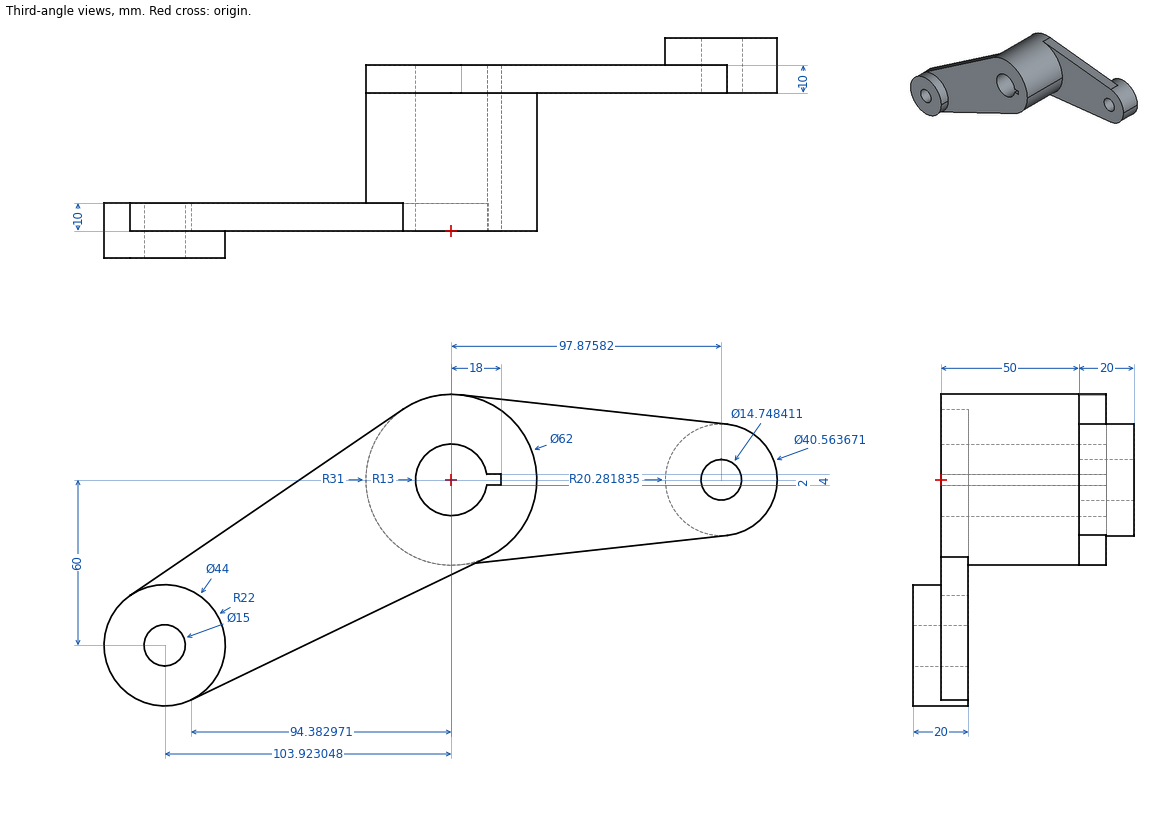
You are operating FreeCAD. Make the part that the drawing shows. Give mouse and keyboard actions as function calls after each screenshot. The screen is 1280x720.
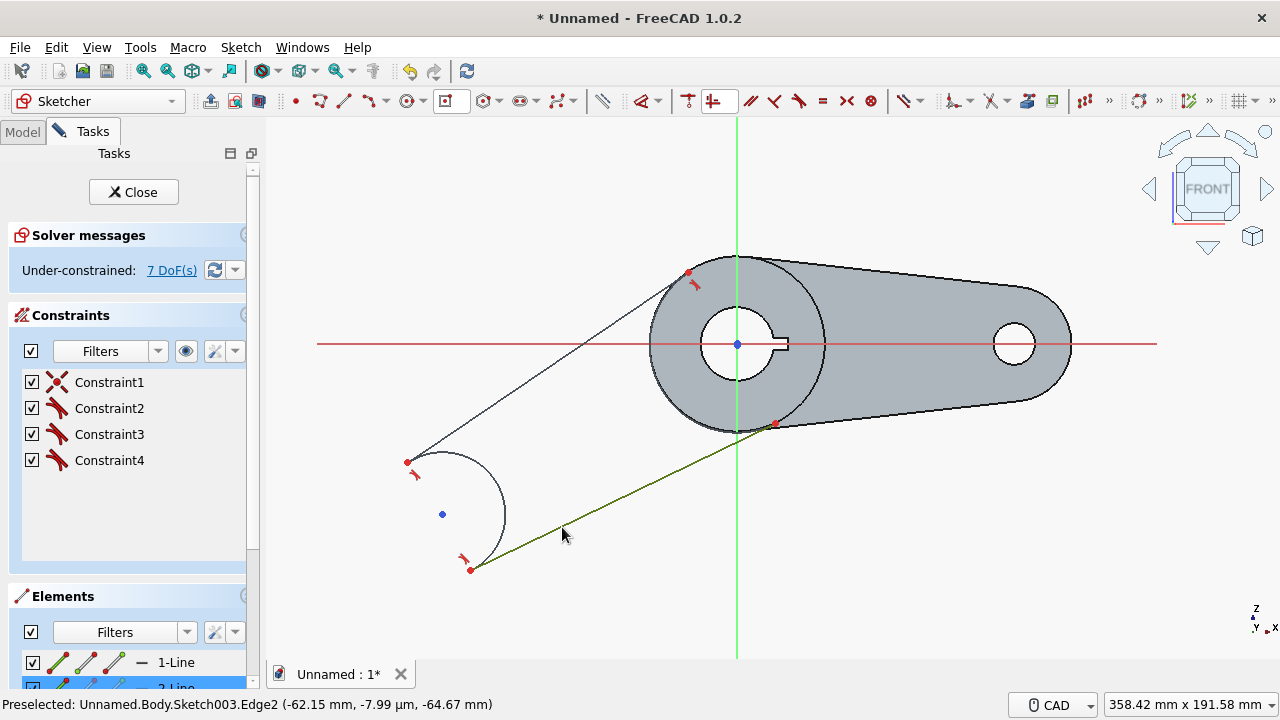
click(699, 424)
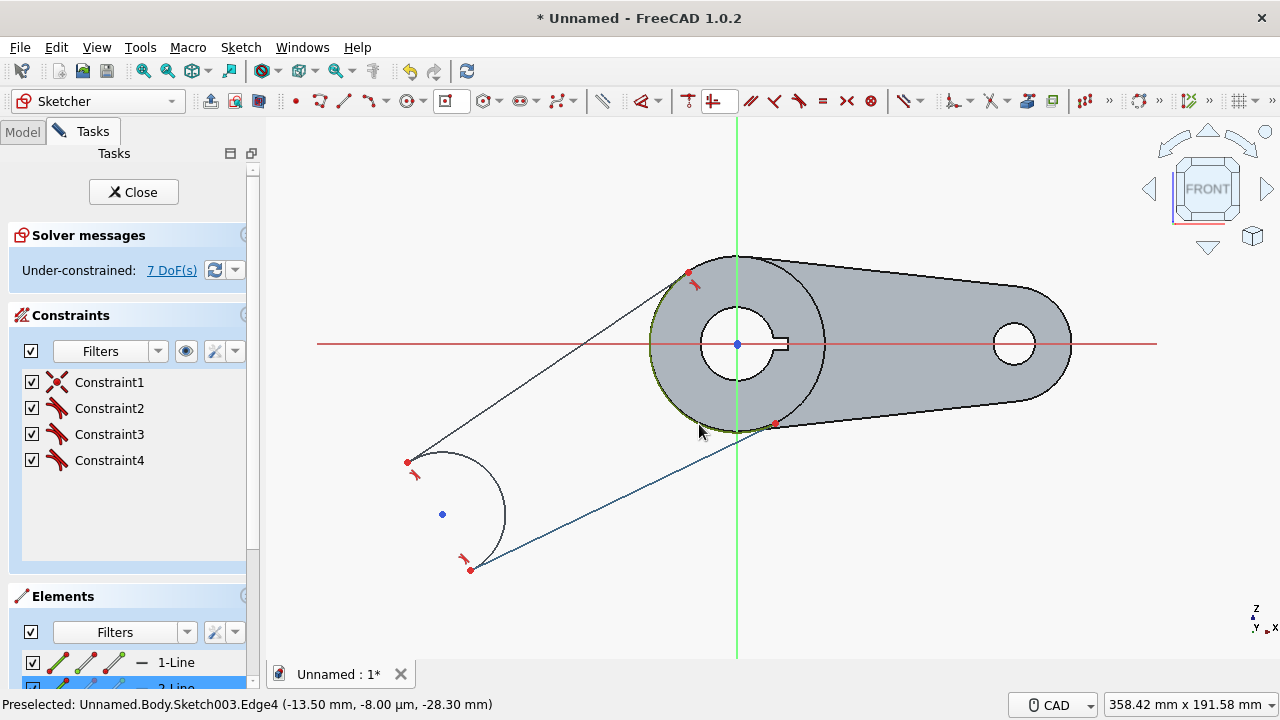
click(800, 102)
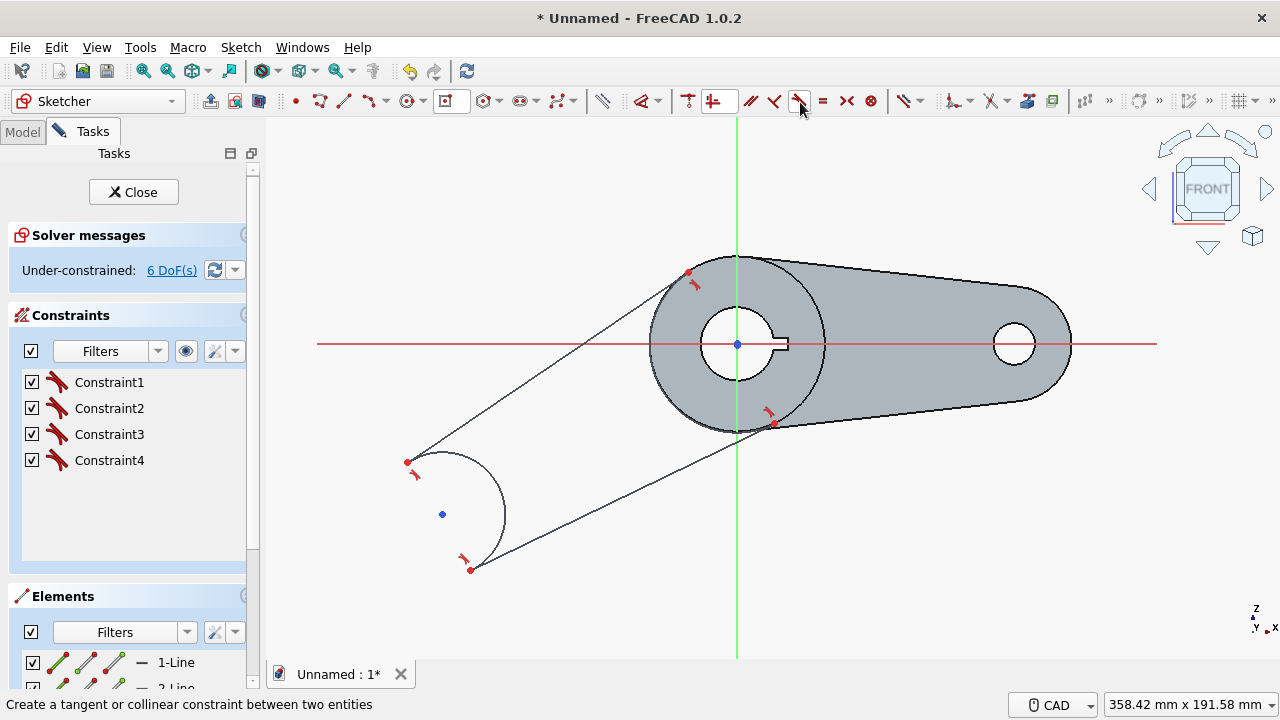
drag(727, 334, 747, 355)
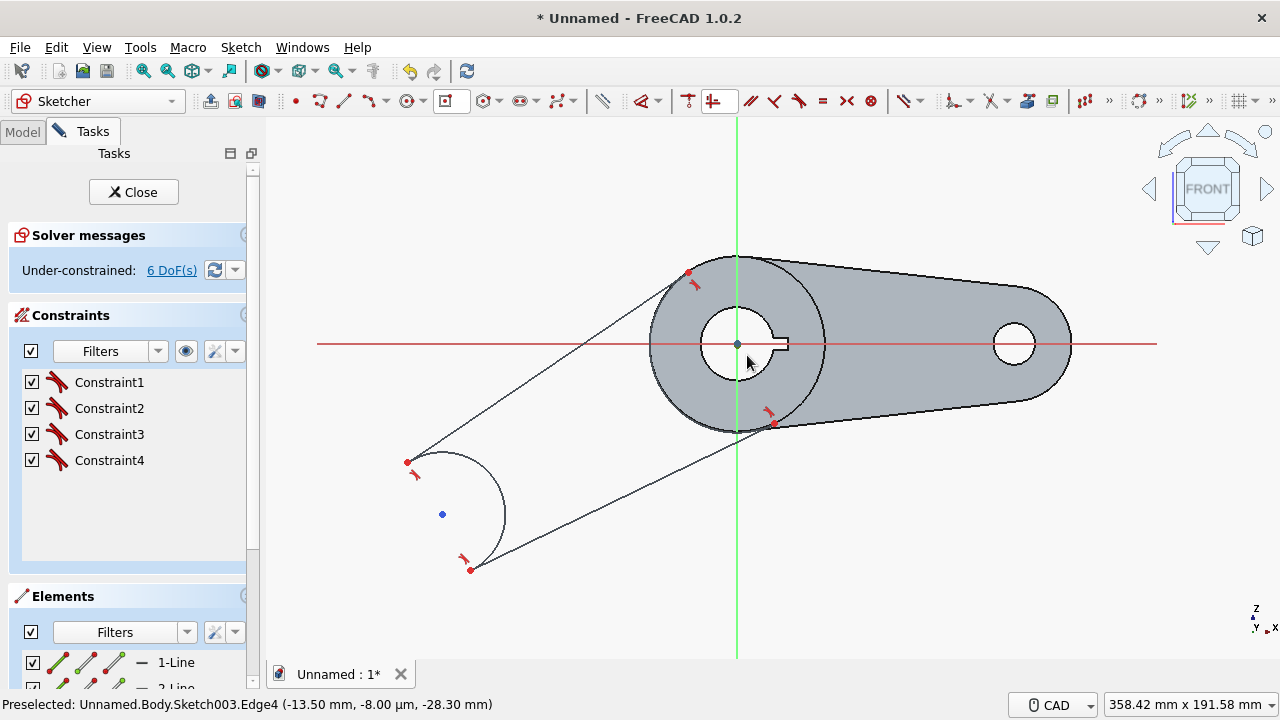
click(688, 102)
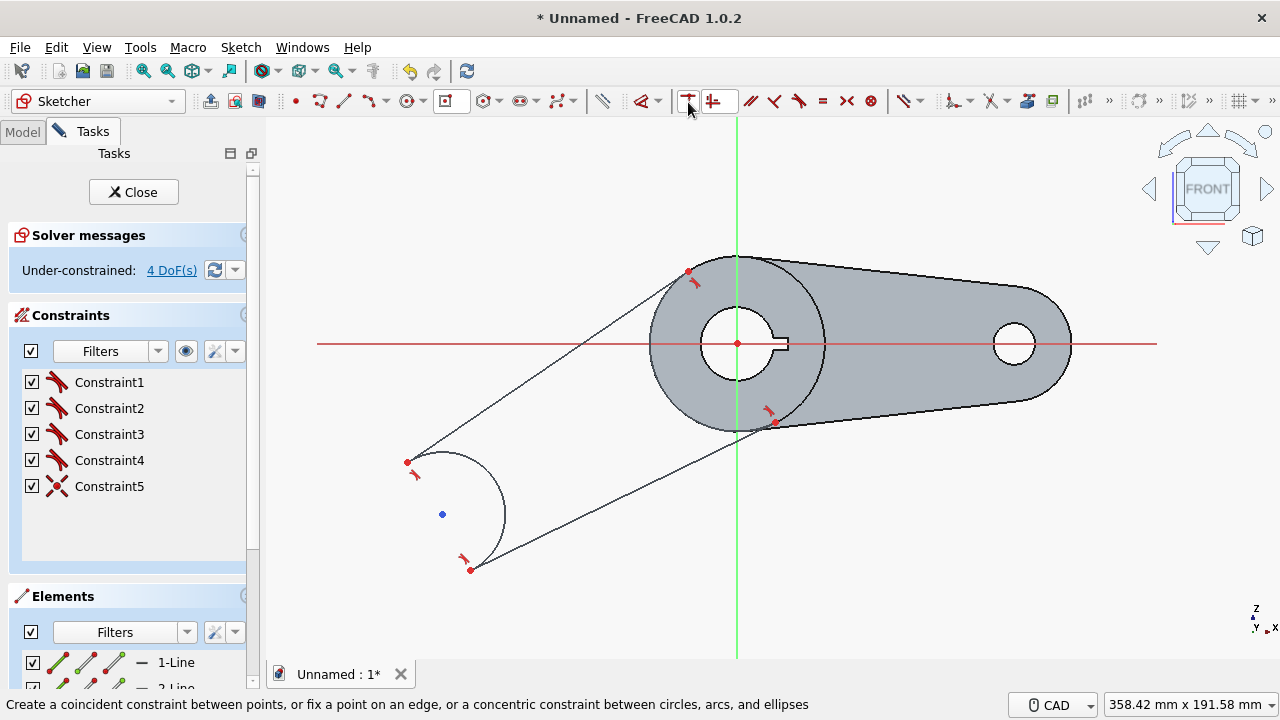
click(642, 102)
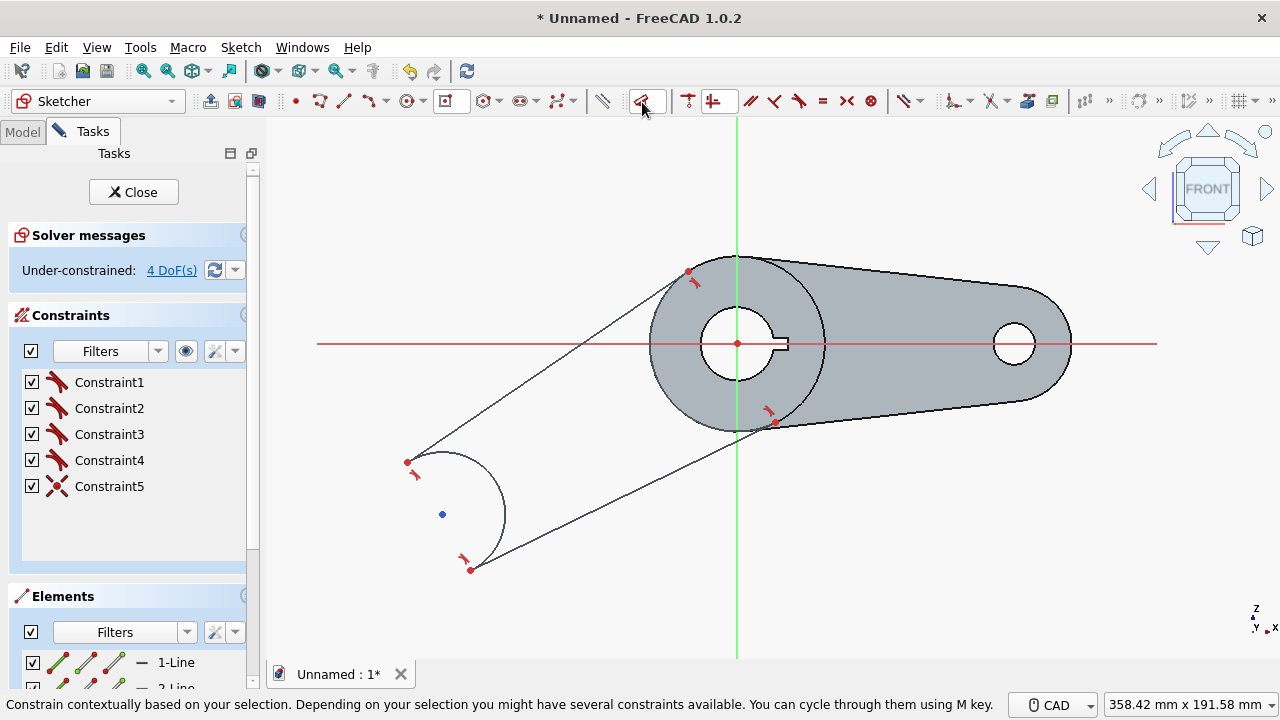
click(505, 523)
click(519, 571)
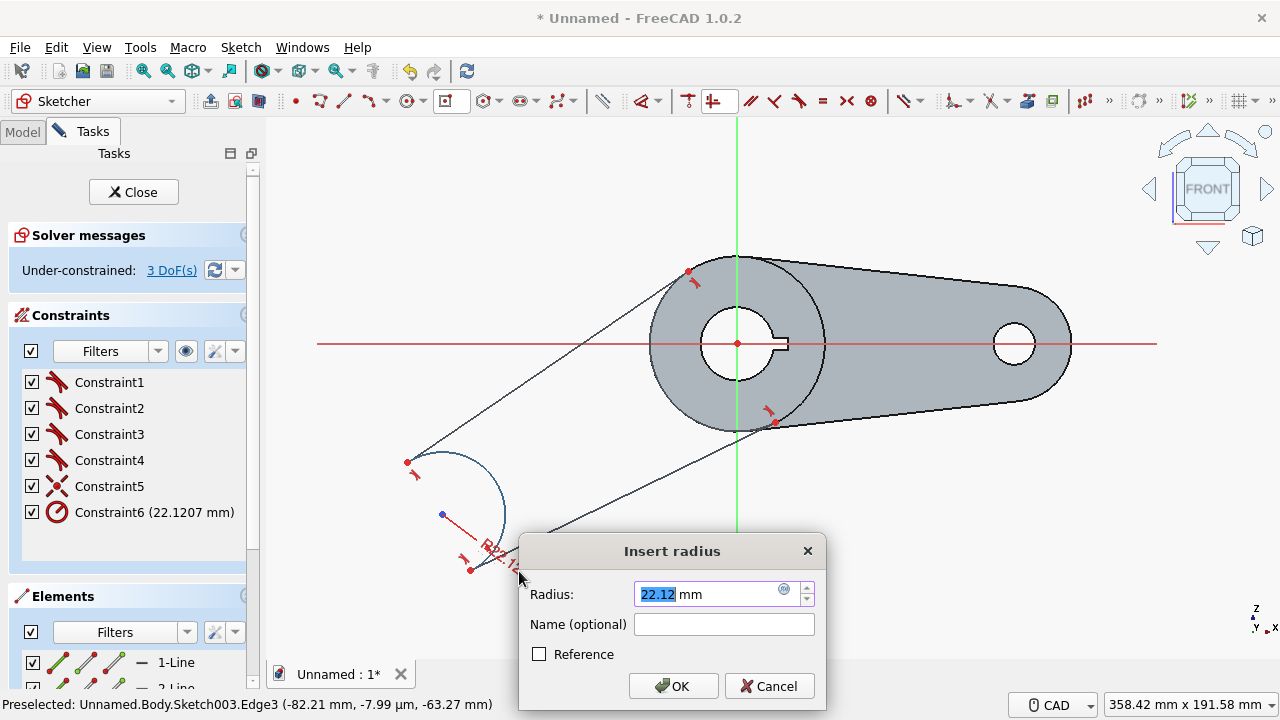
text(22)
key(Return)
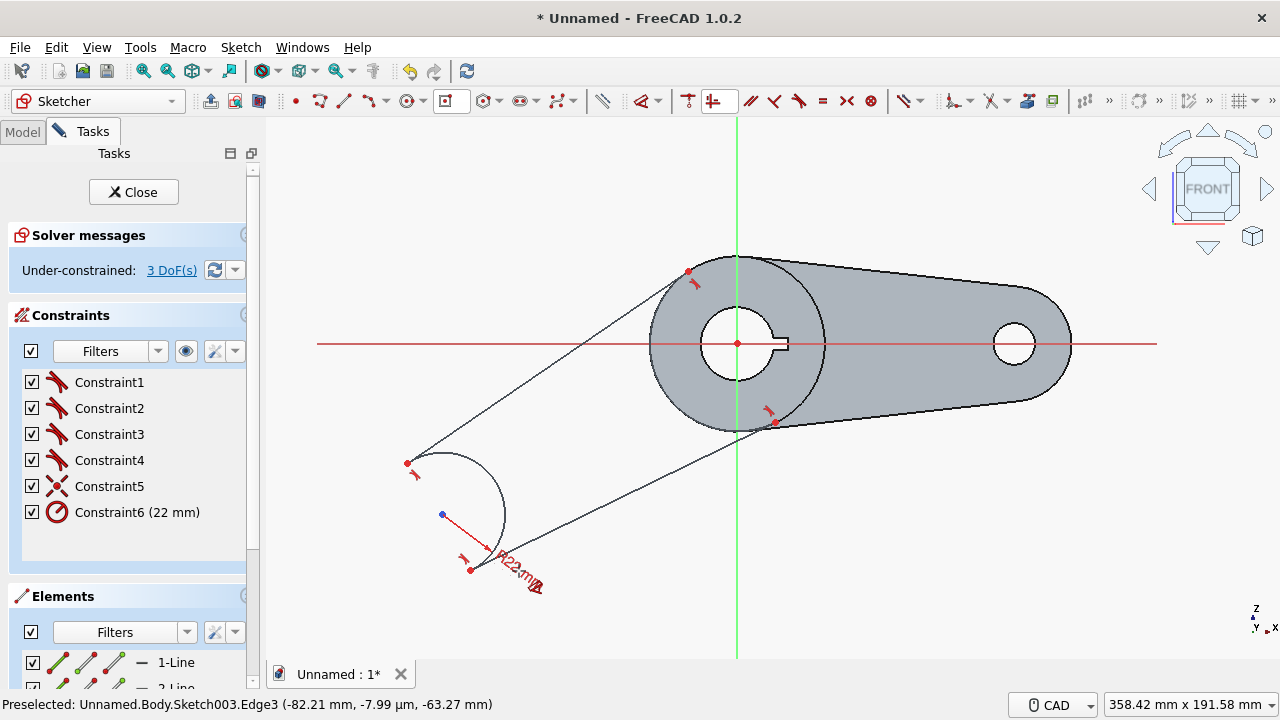
click(700, 423)
click(641, 414)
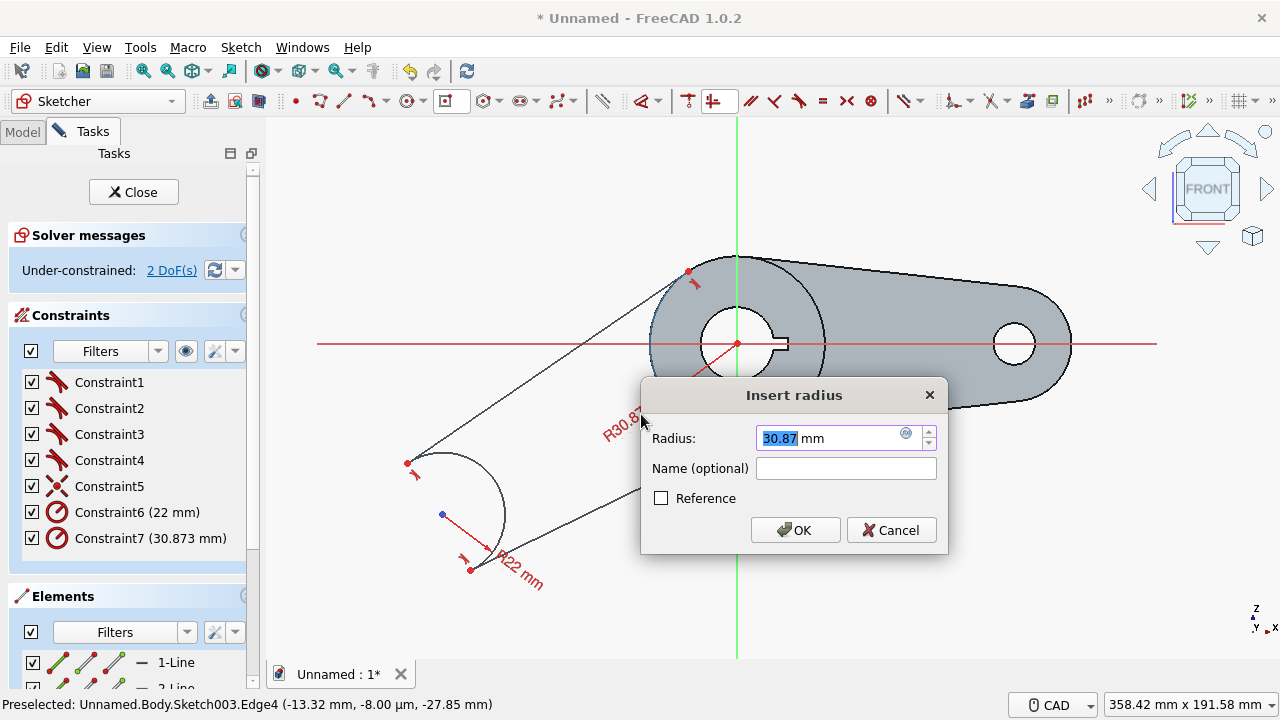
text(31)
key(Return)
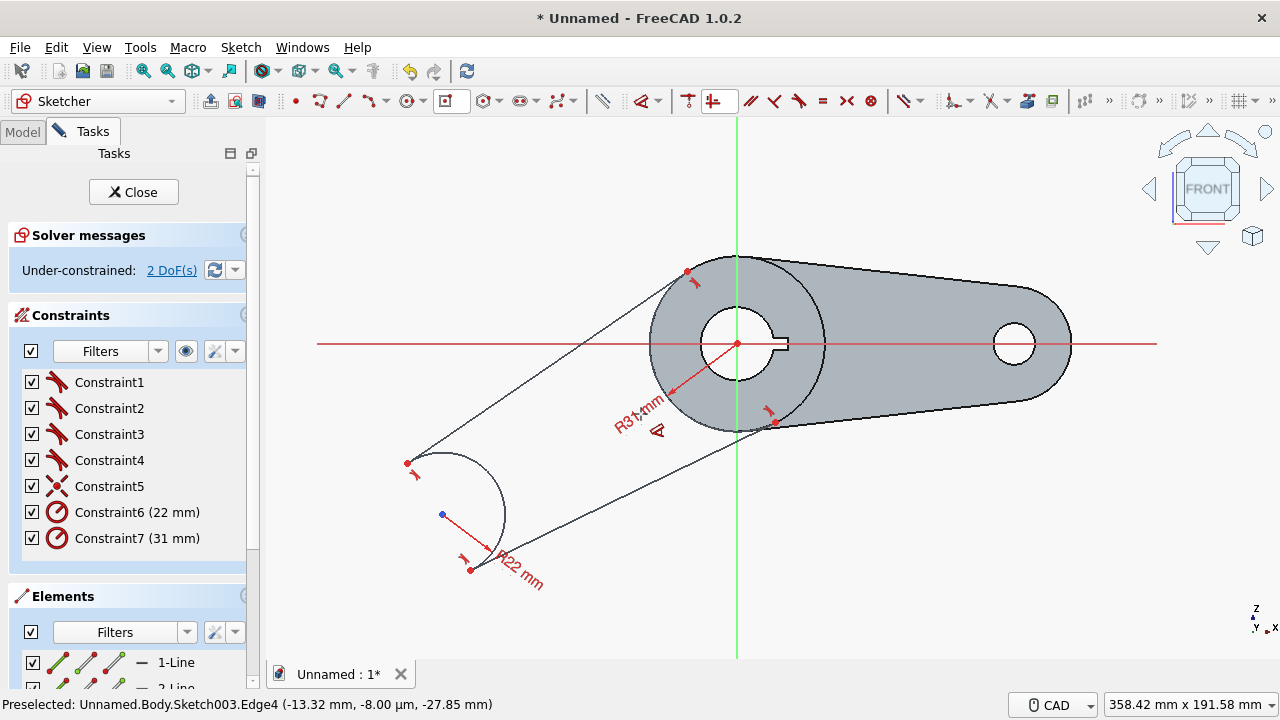
click(443, 515)
click(409, 429)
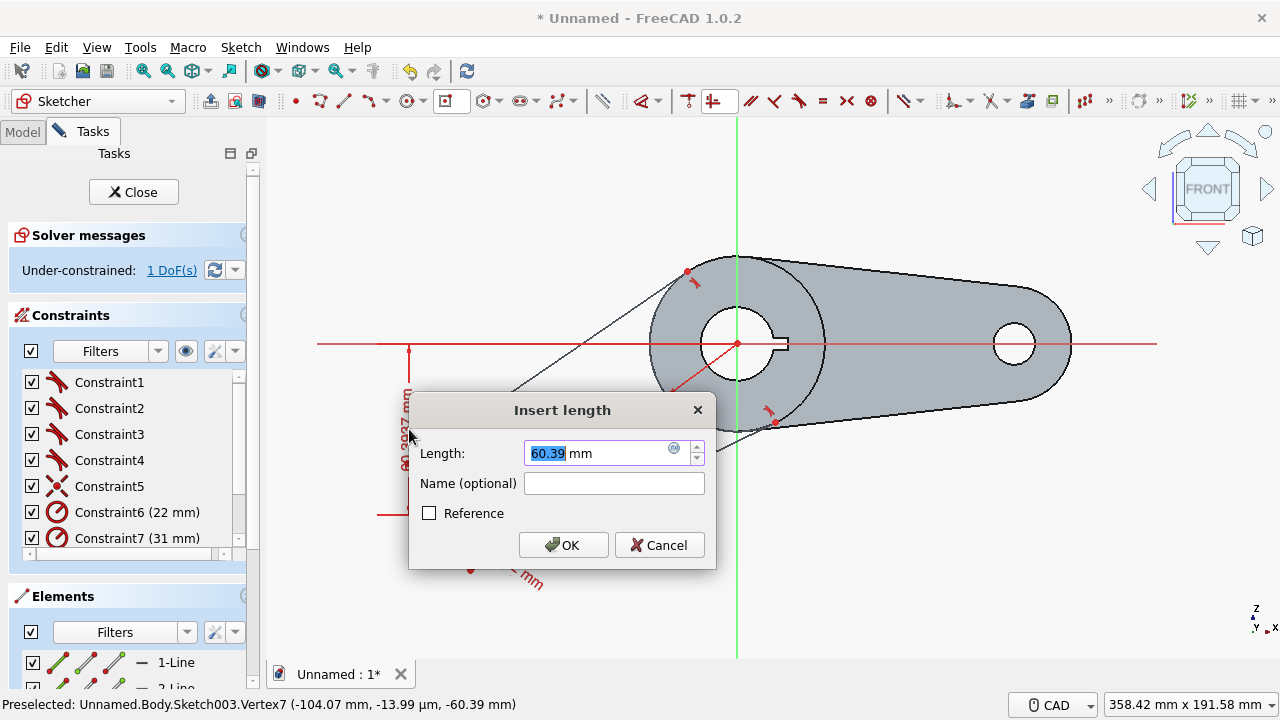
text(60)
key(Return)